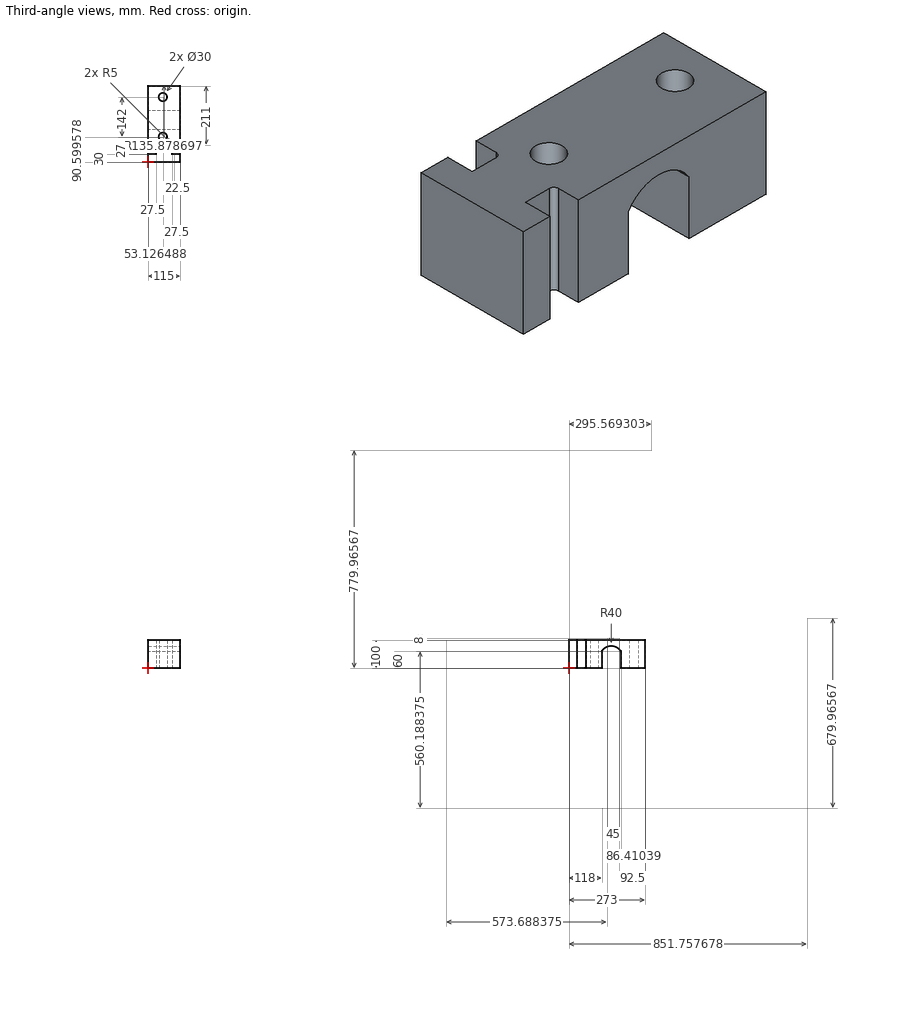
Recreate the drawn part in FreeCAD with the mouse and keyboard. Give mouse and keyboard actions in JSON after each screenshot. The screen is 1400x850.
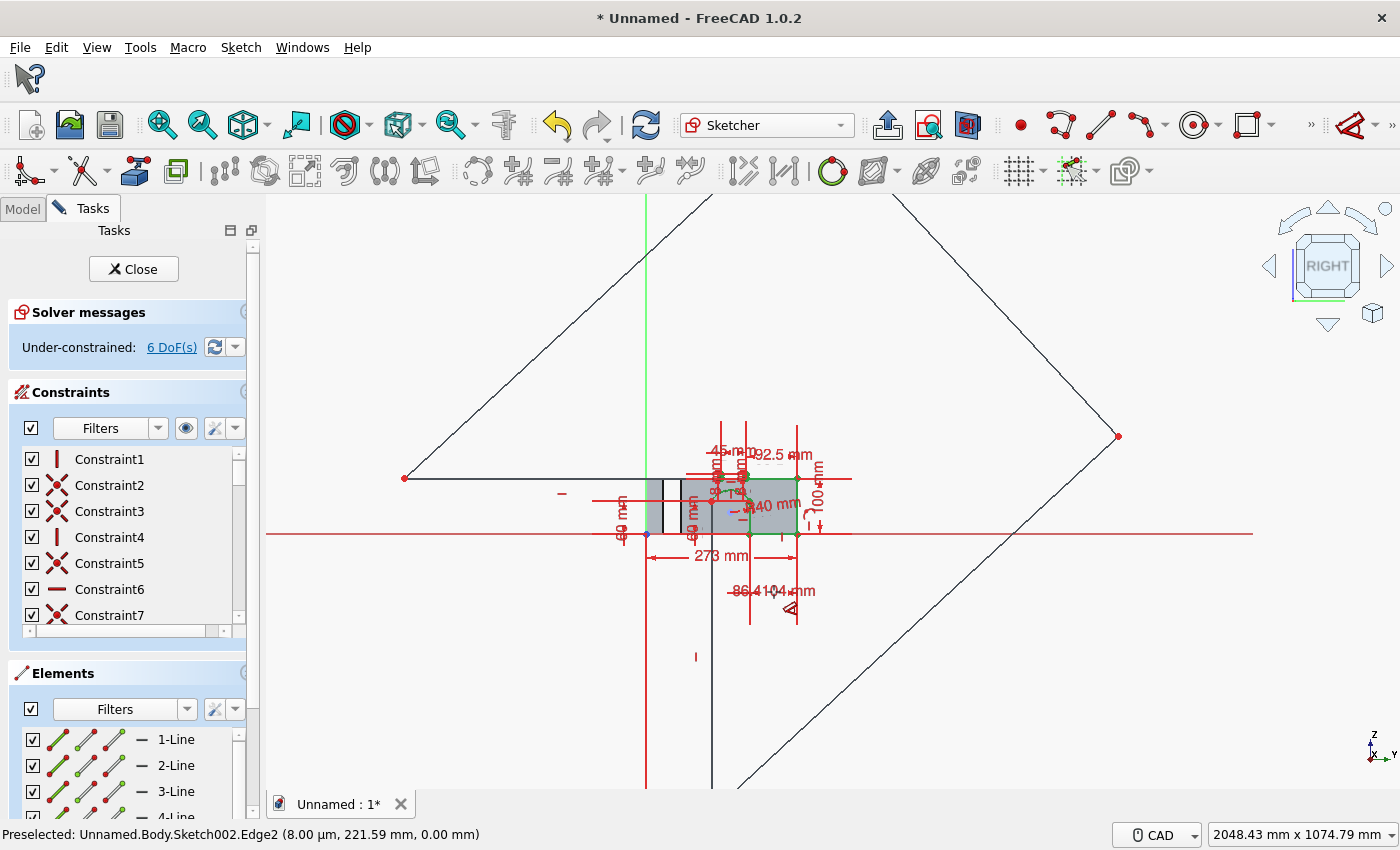
{"action": "left_click", "coordinate": [626, 479]}
{"action": "left_click", "coordinate": [490, 513]}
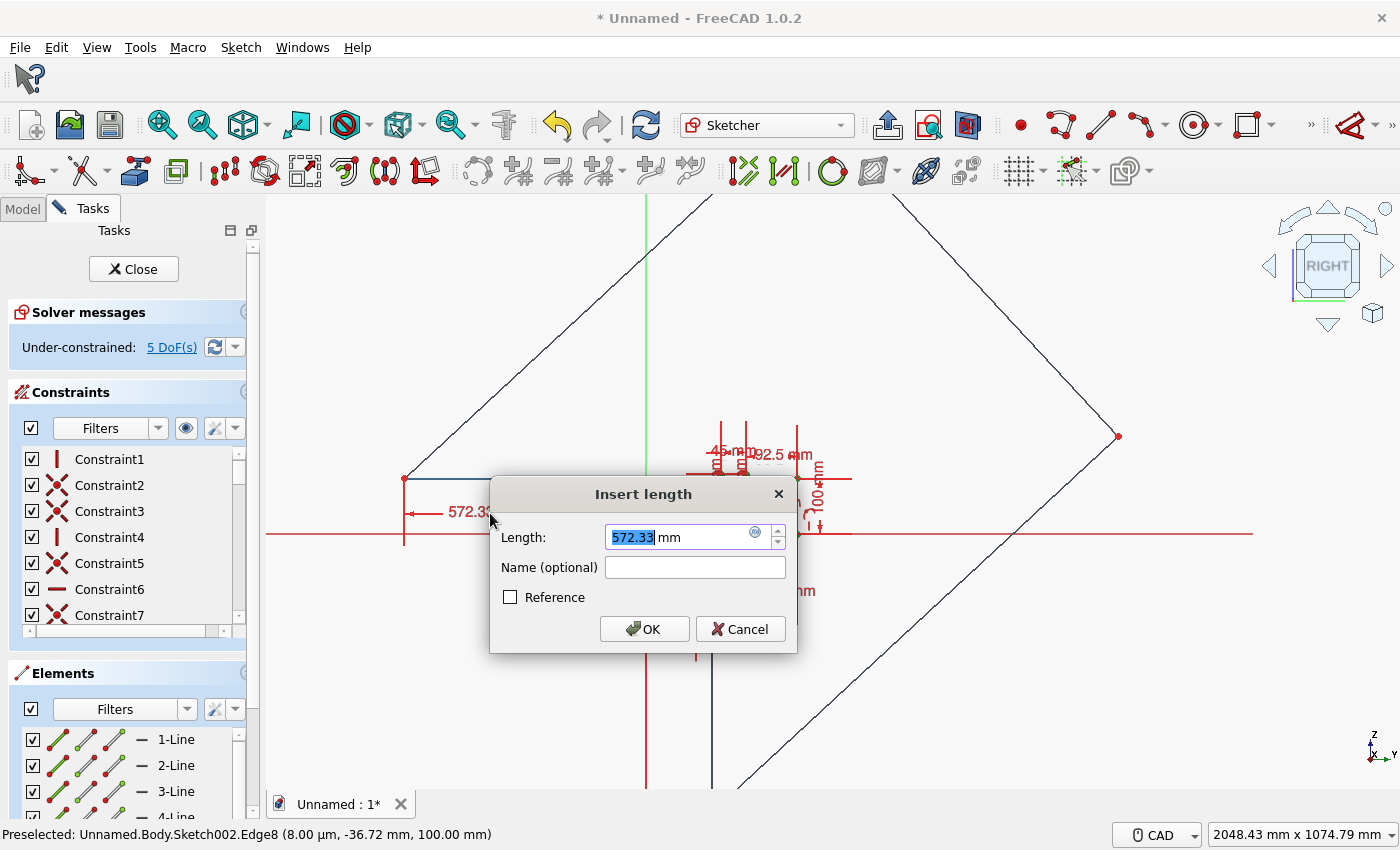
{"action": "type", "text": "573.688375"}
{"action": "key", "text": "Return"}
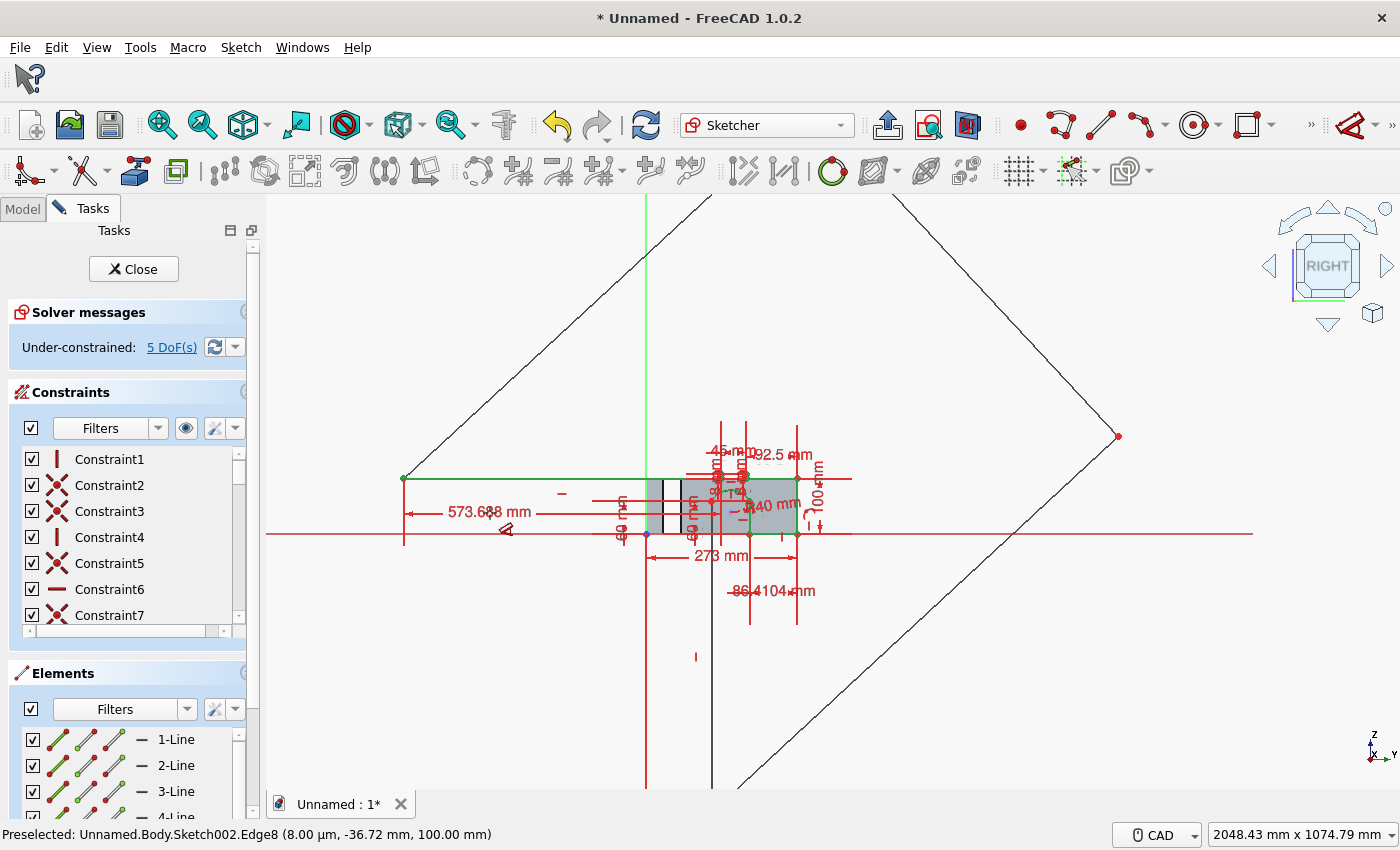
{"action": "left_click", "coordinate": [712, 719]}
{"action": "left_click", "coordinate": [678, 631]}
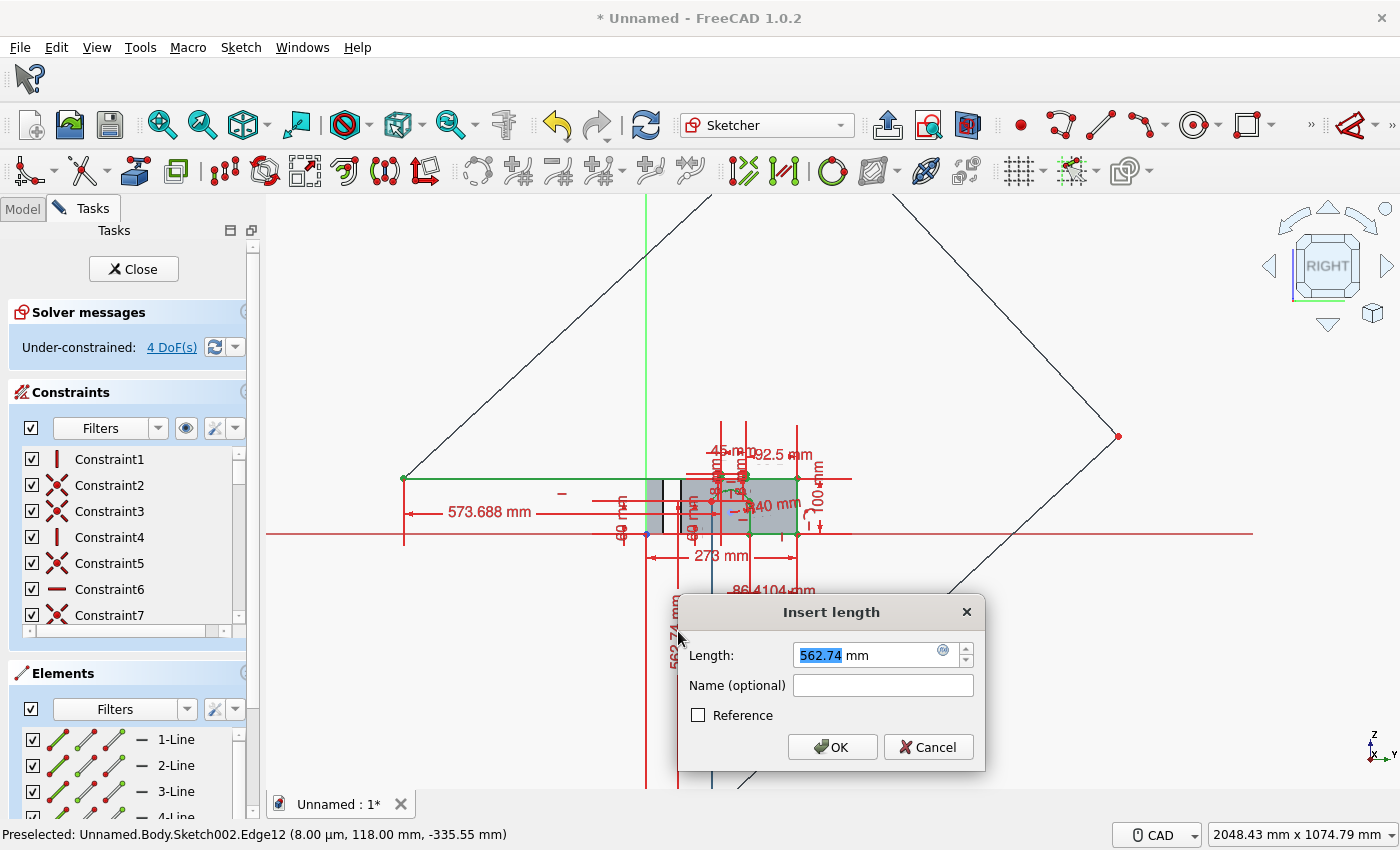
{"action": "type", "text": "560.188375"}
{"action": "key", "text": "Return"}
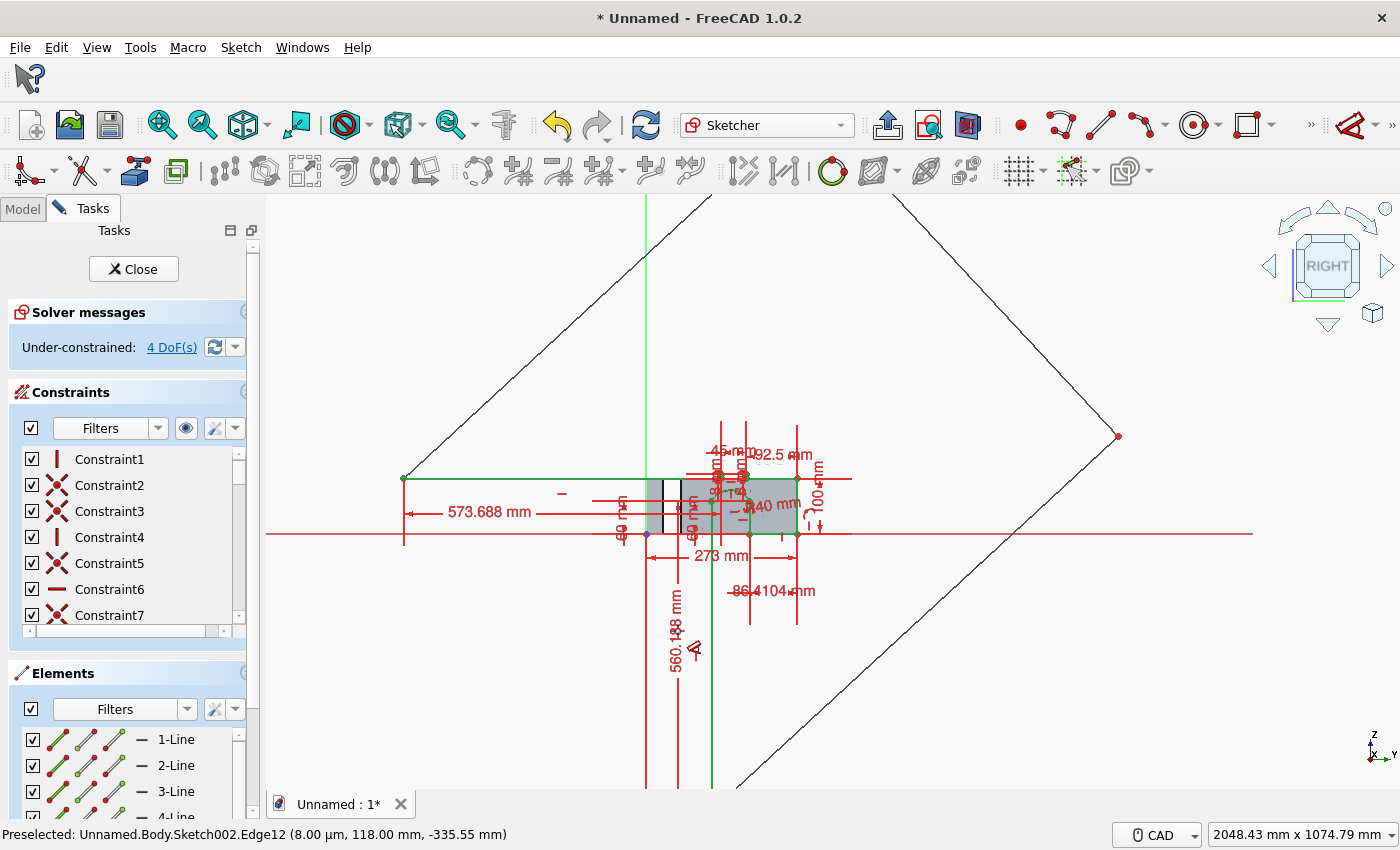
{"action": "scroll", "coordinate": [769, 534], "scroll_direction": "down", "scroll_amount": 3}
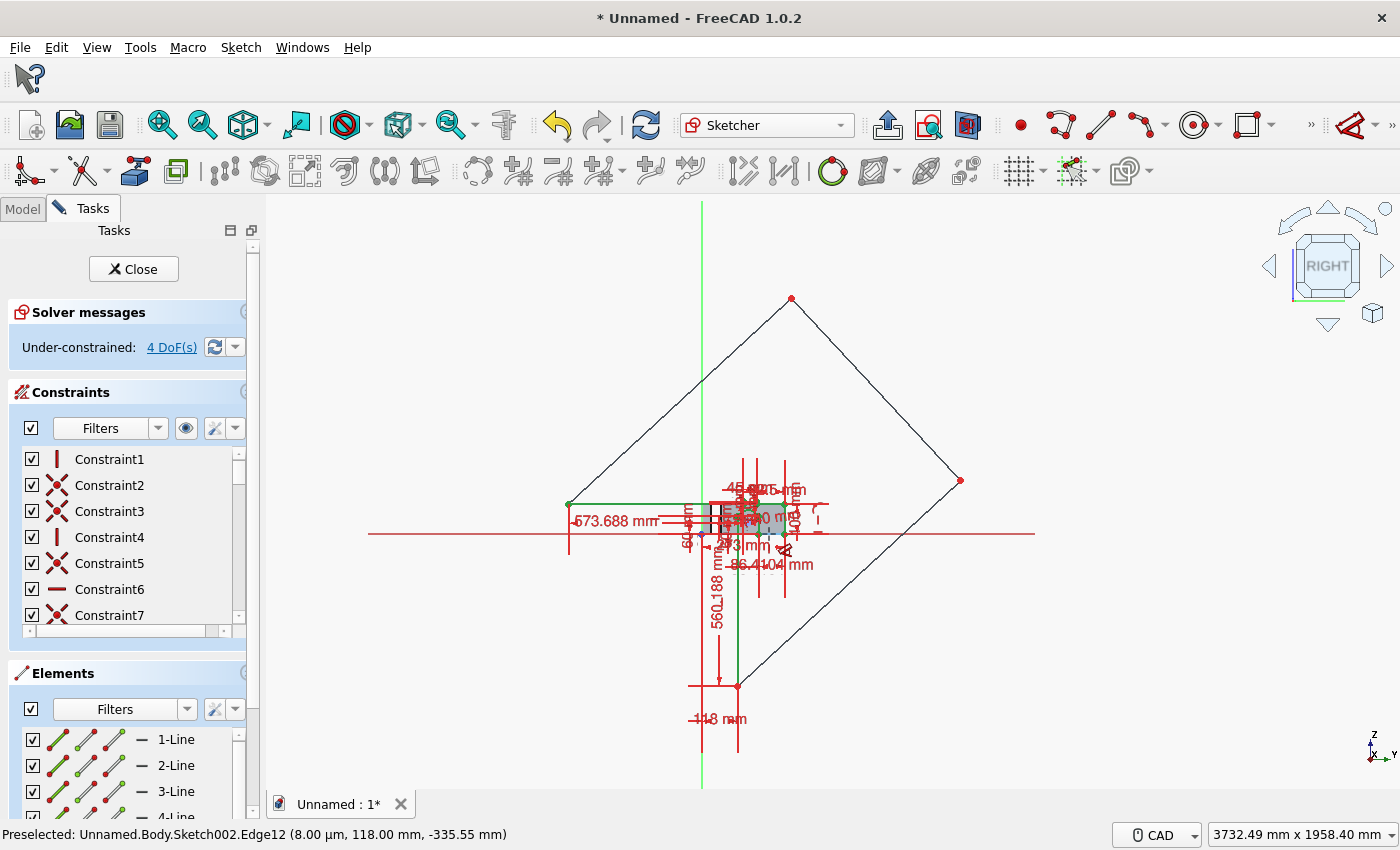
{"action": "left_click", "coordinate": [791, 298]}
{"action": "left_click", "coordinate": [668, 362]}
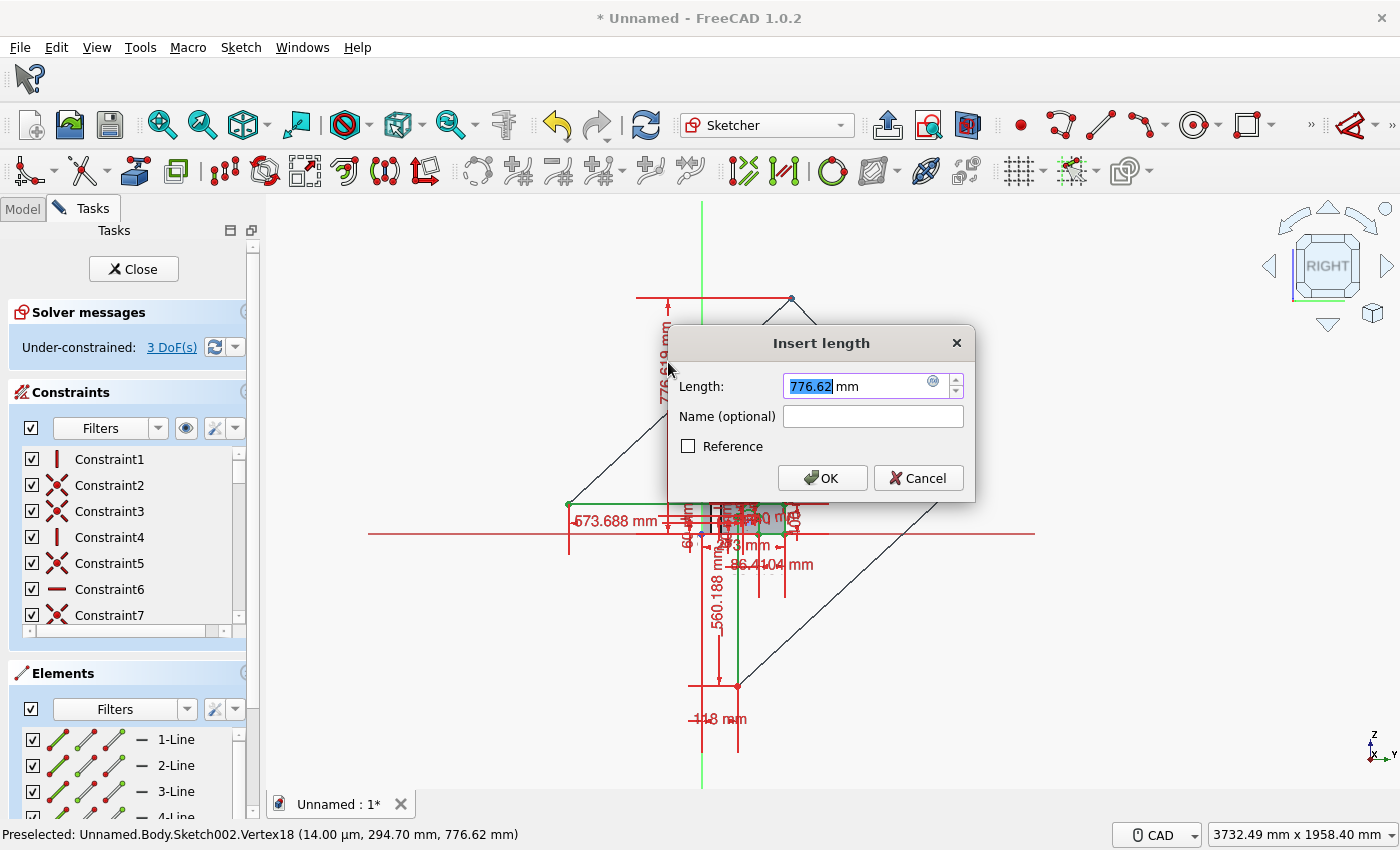
{"action": "type", "text": "779.96567"}
{"action": "key", "text": "Return"}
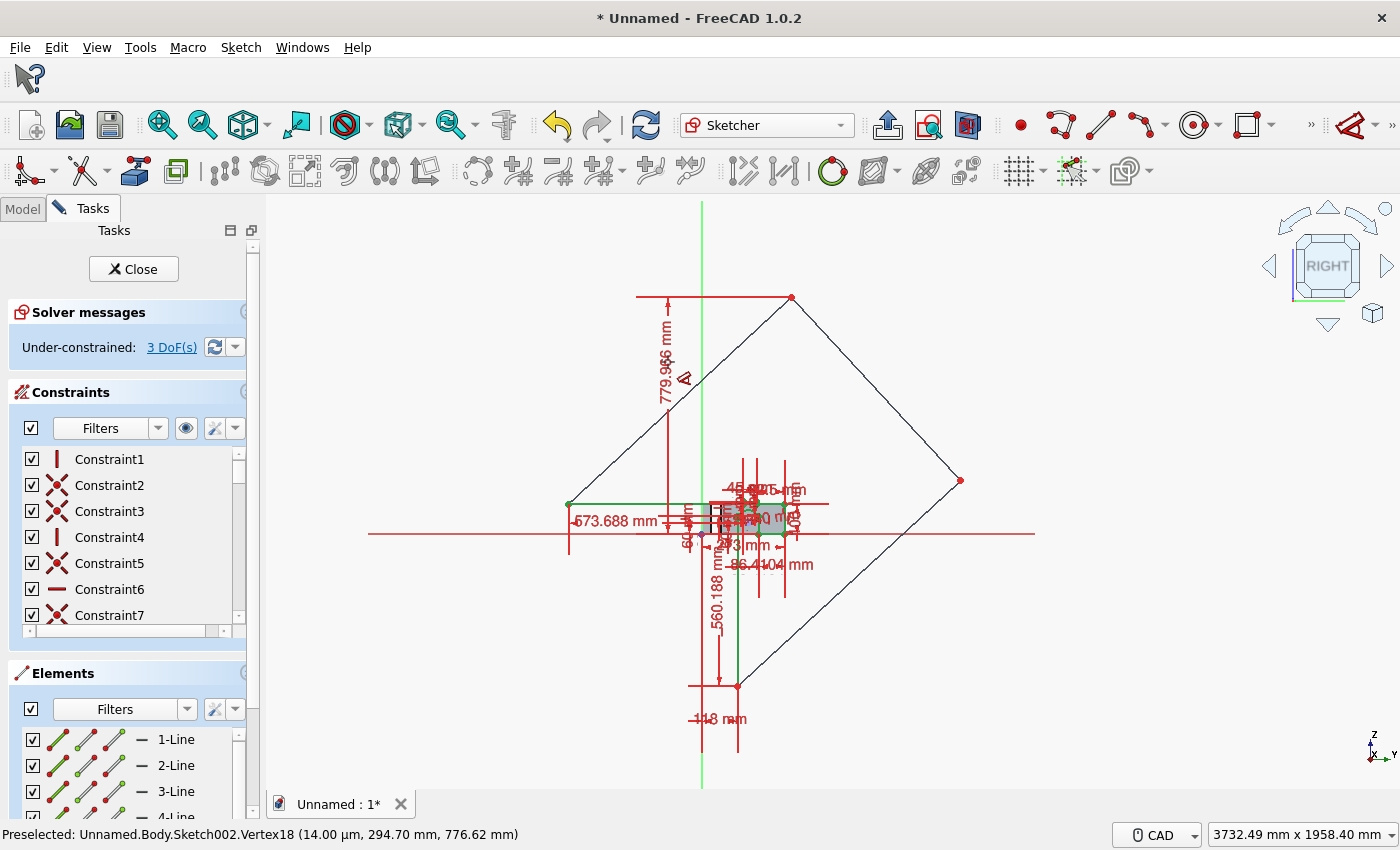
{"action": "left_click", "coordinate": [805, 625]}
{"action": "left_click", "coordinate": [995, 584]}